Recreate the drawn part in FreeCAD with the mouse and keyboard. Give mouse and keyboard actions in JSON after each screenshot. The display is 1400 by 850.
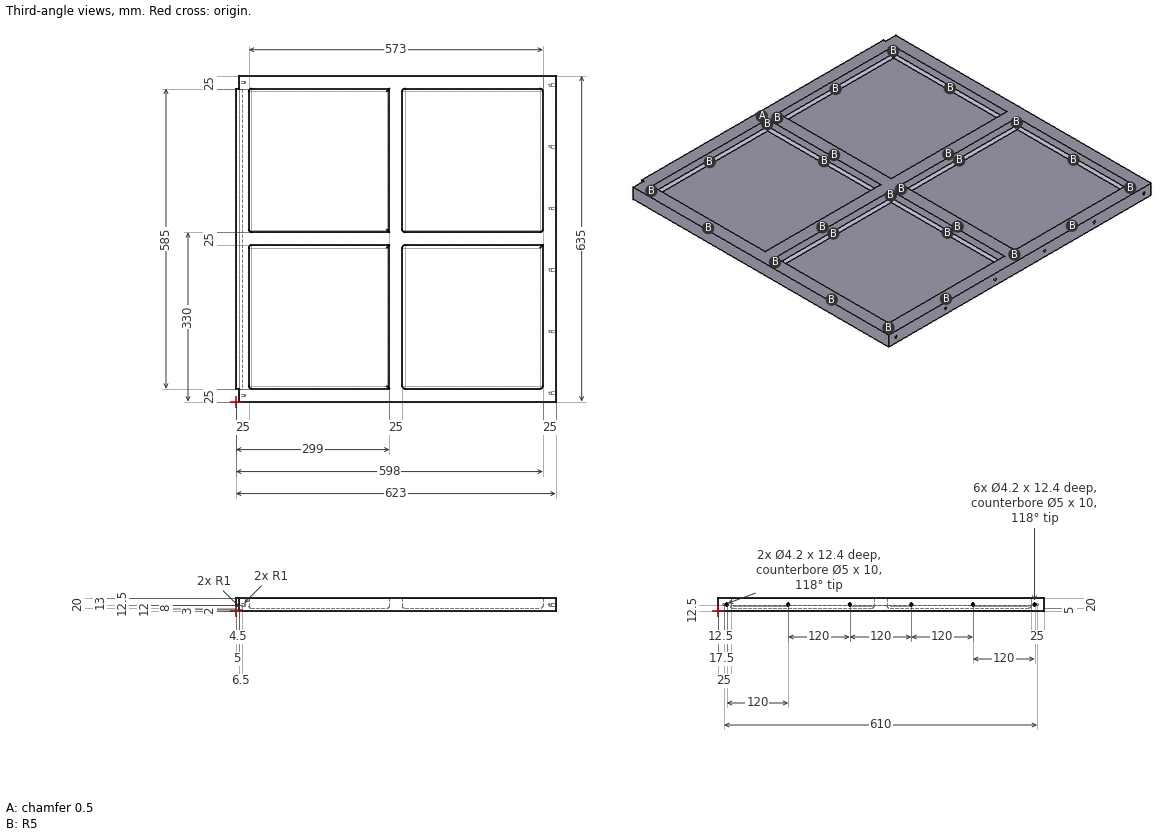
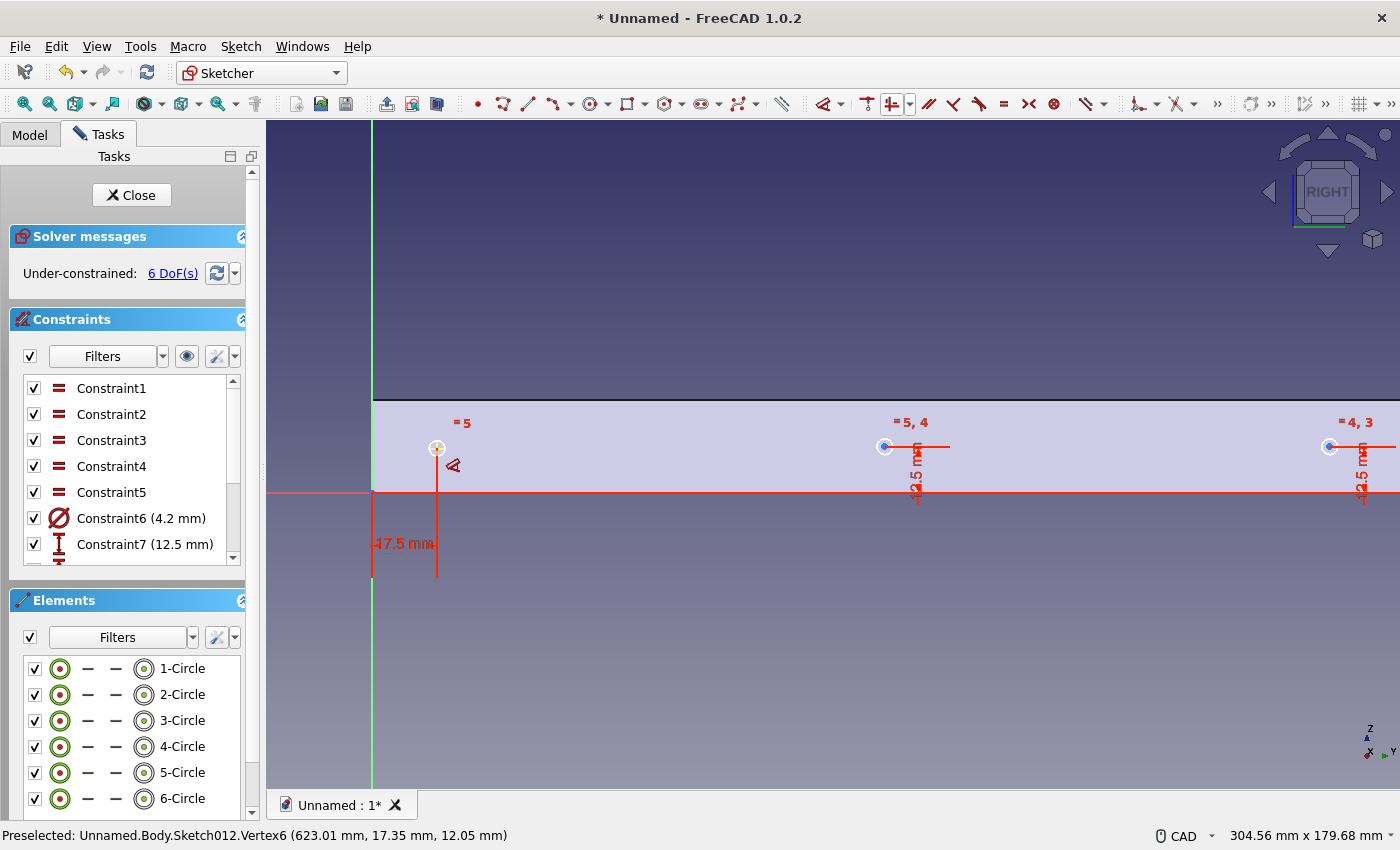
{"action": "left_click", "coordinate": [437, 448]}
{"action": "left_click", "coordinate": [338, 471]}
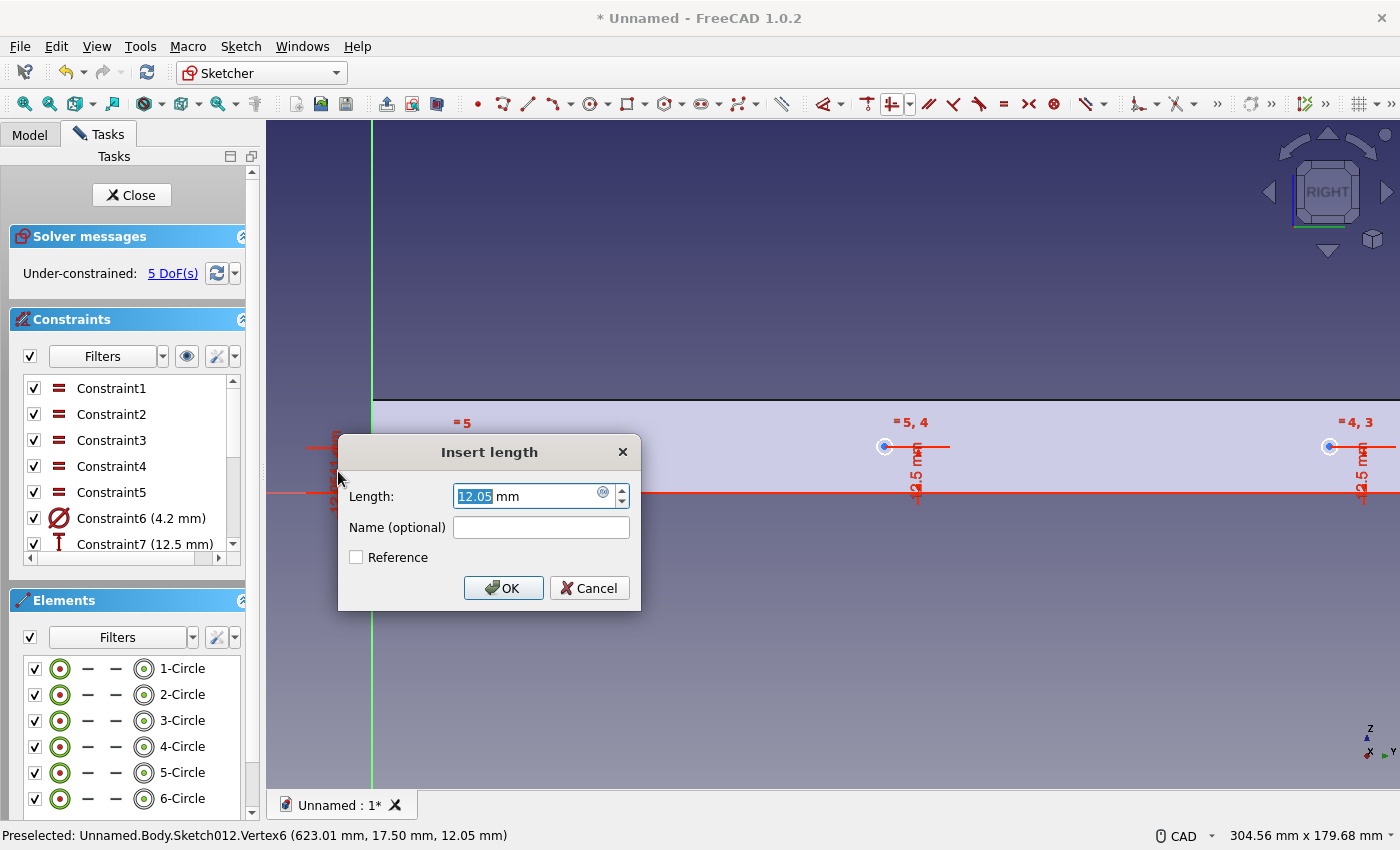
{"action": "type", "text": "12.5"}
{"action": "key", "text": "Return"}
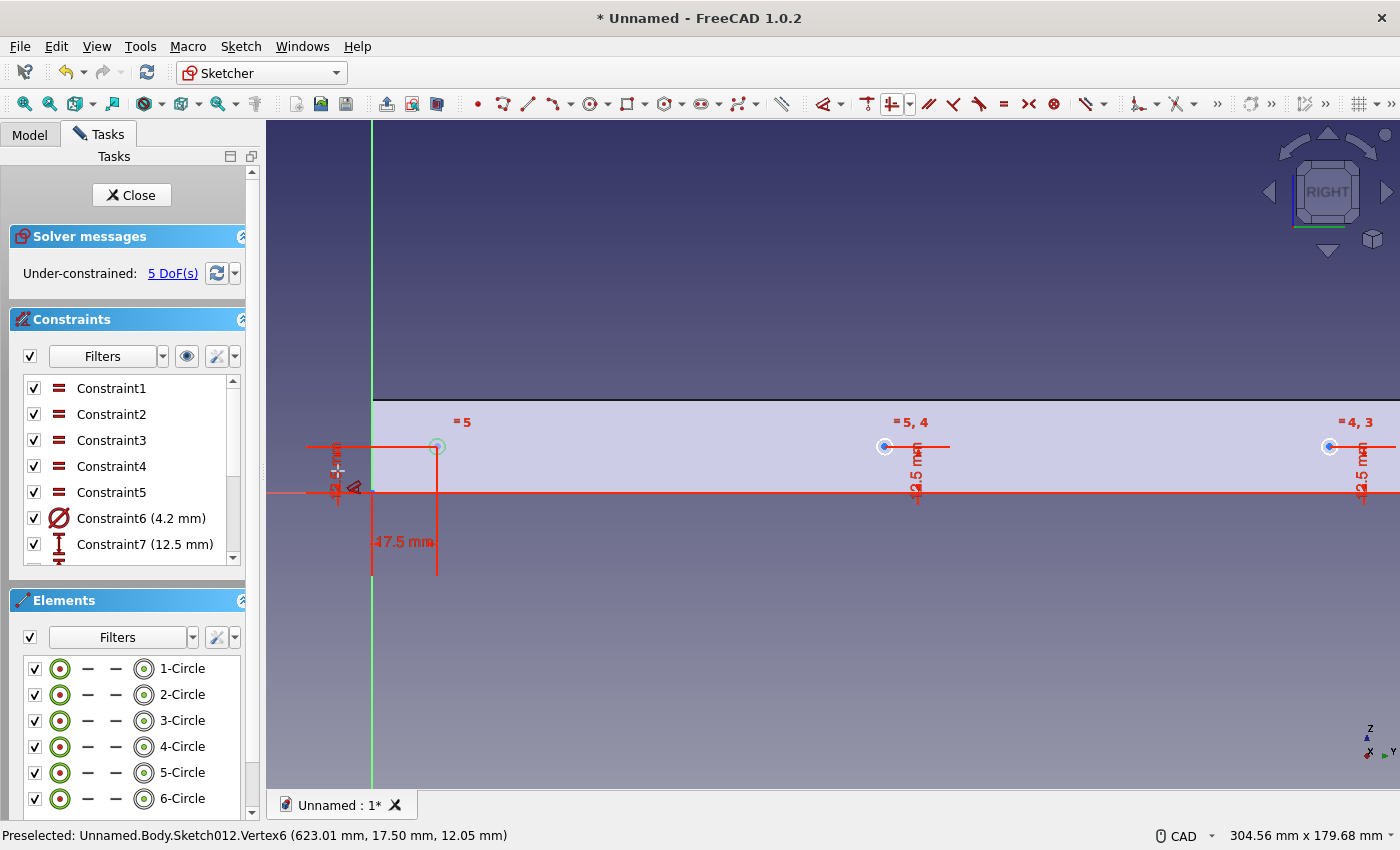
{"action": "scroll", "coordinate": [436, 449], "scroll_direction": "down", "scroll_amount": 6}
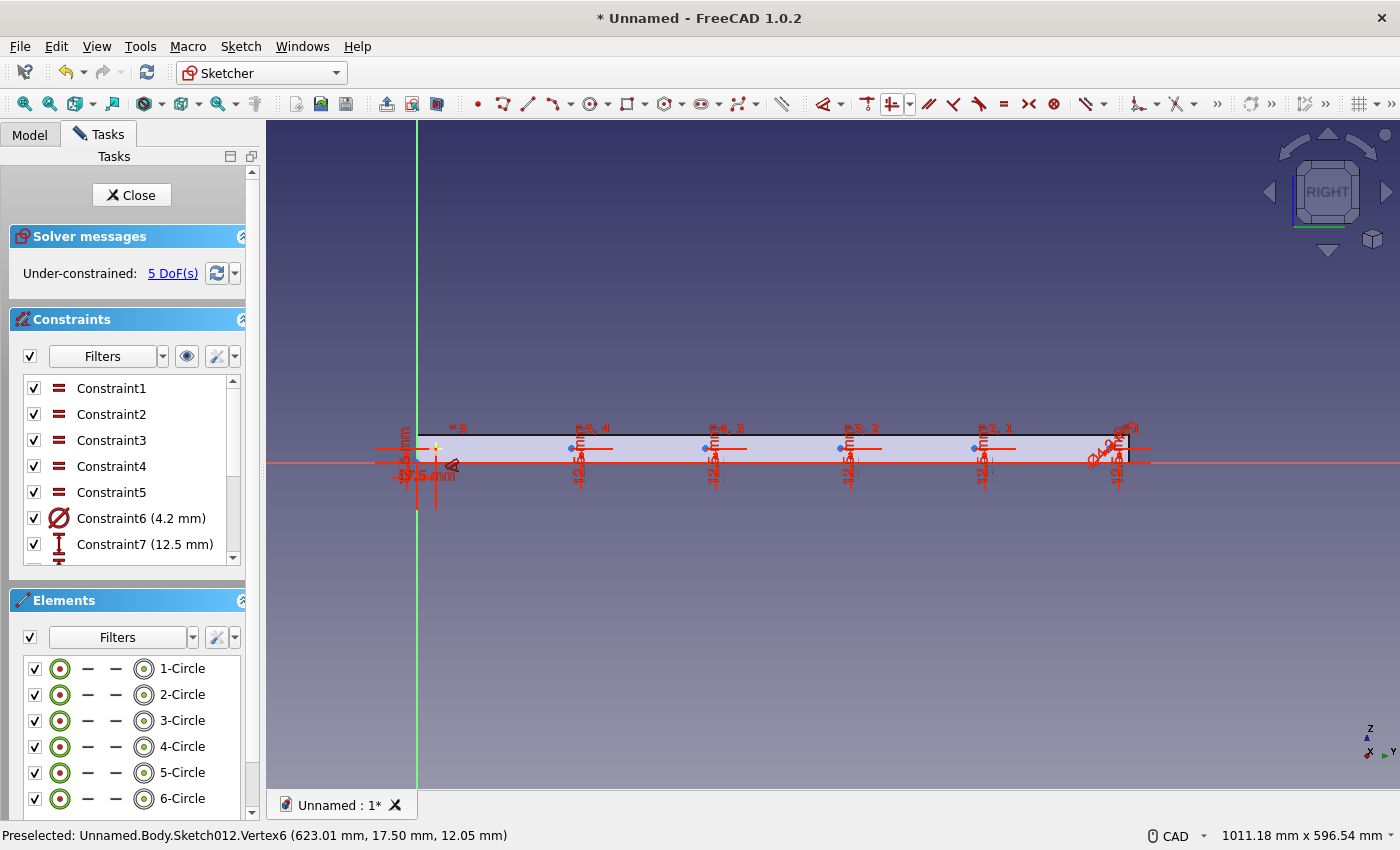
{"action": "left_click", "coordinate": [1109, 449]}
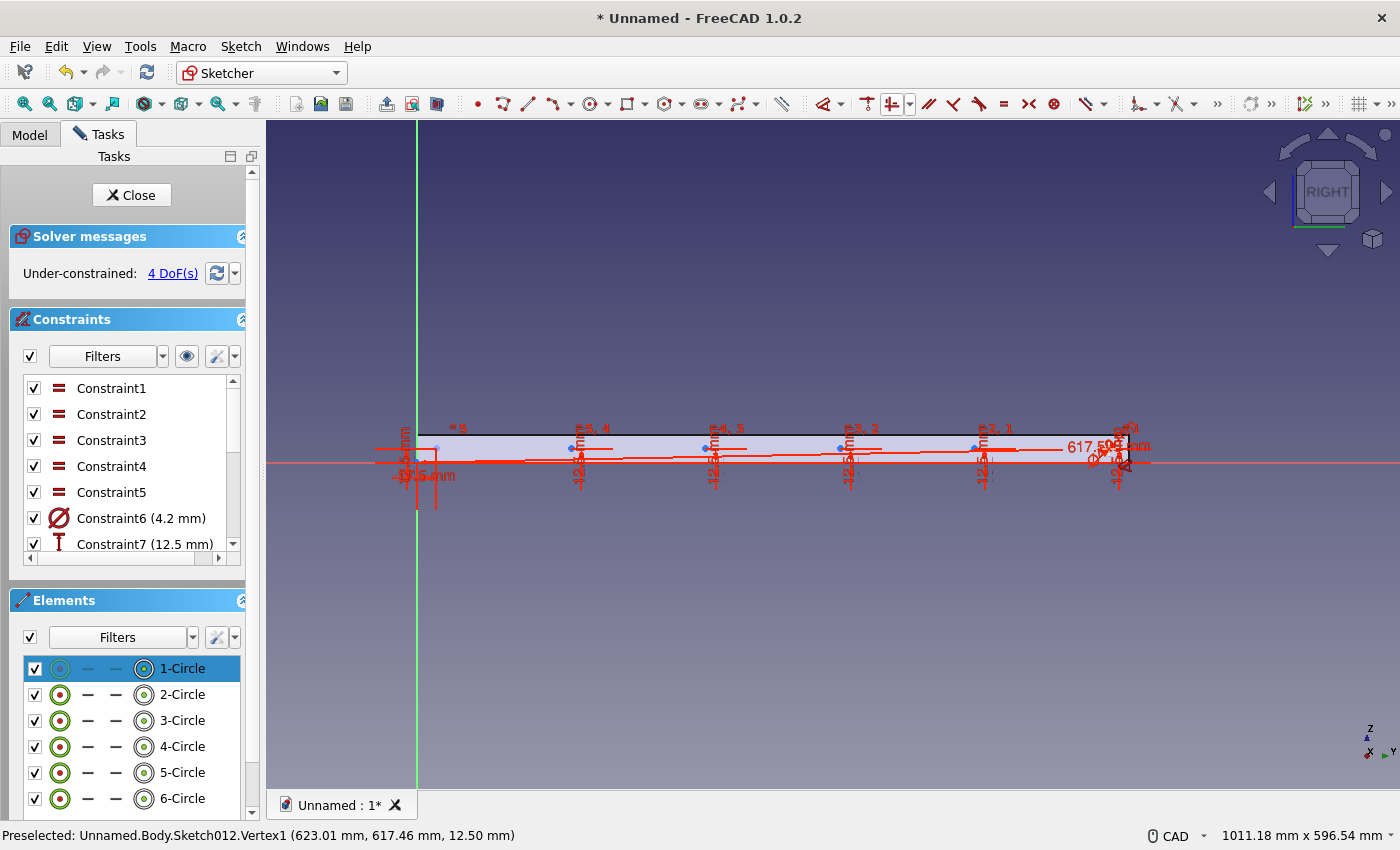
{"action": "left_click", "coordinate": [974, 449]}
{"action": "left_click", "coordinate": [1042, 415]}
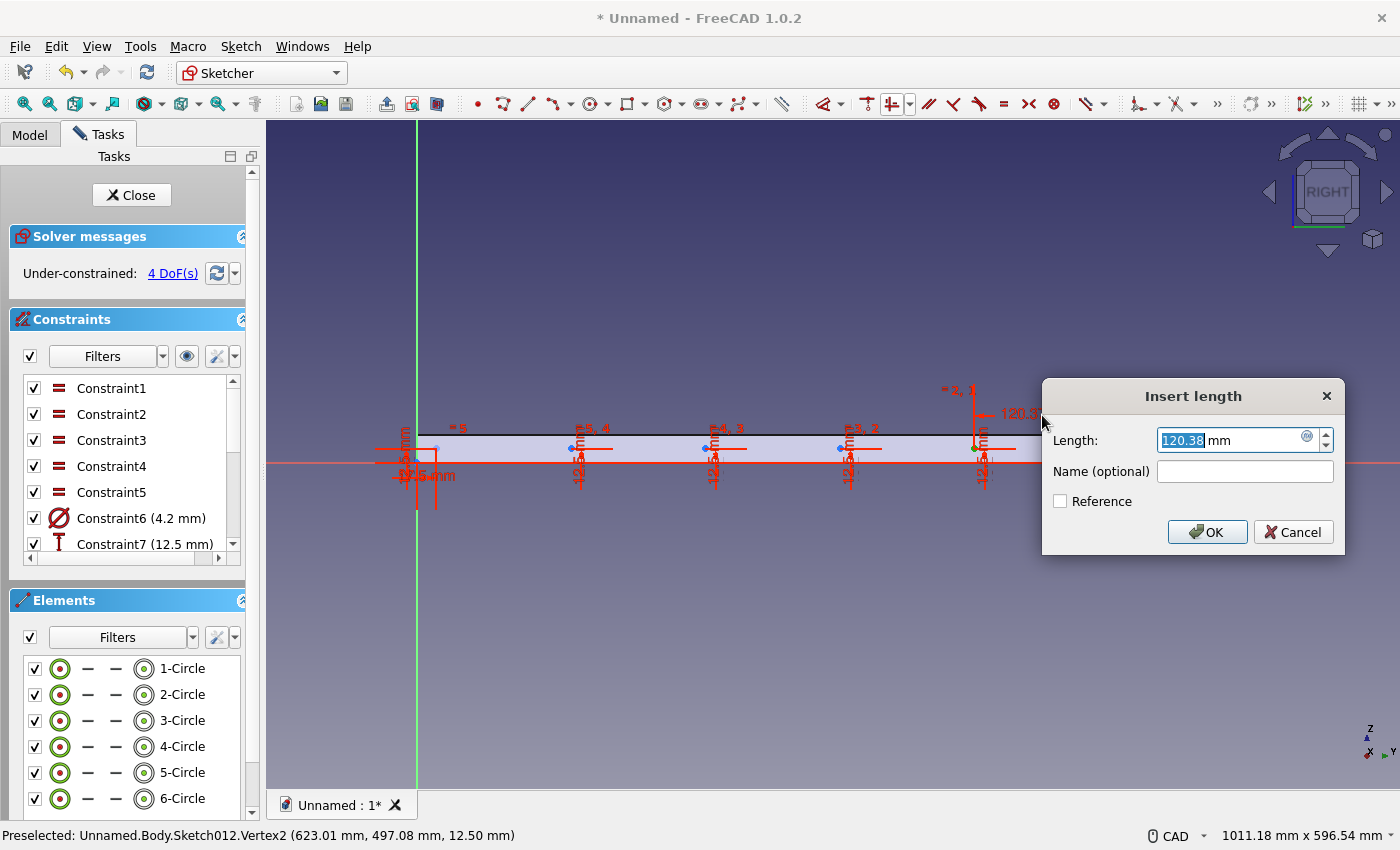
{"action": "type", "text": "120"}
{"action": "key", "text": "Return"}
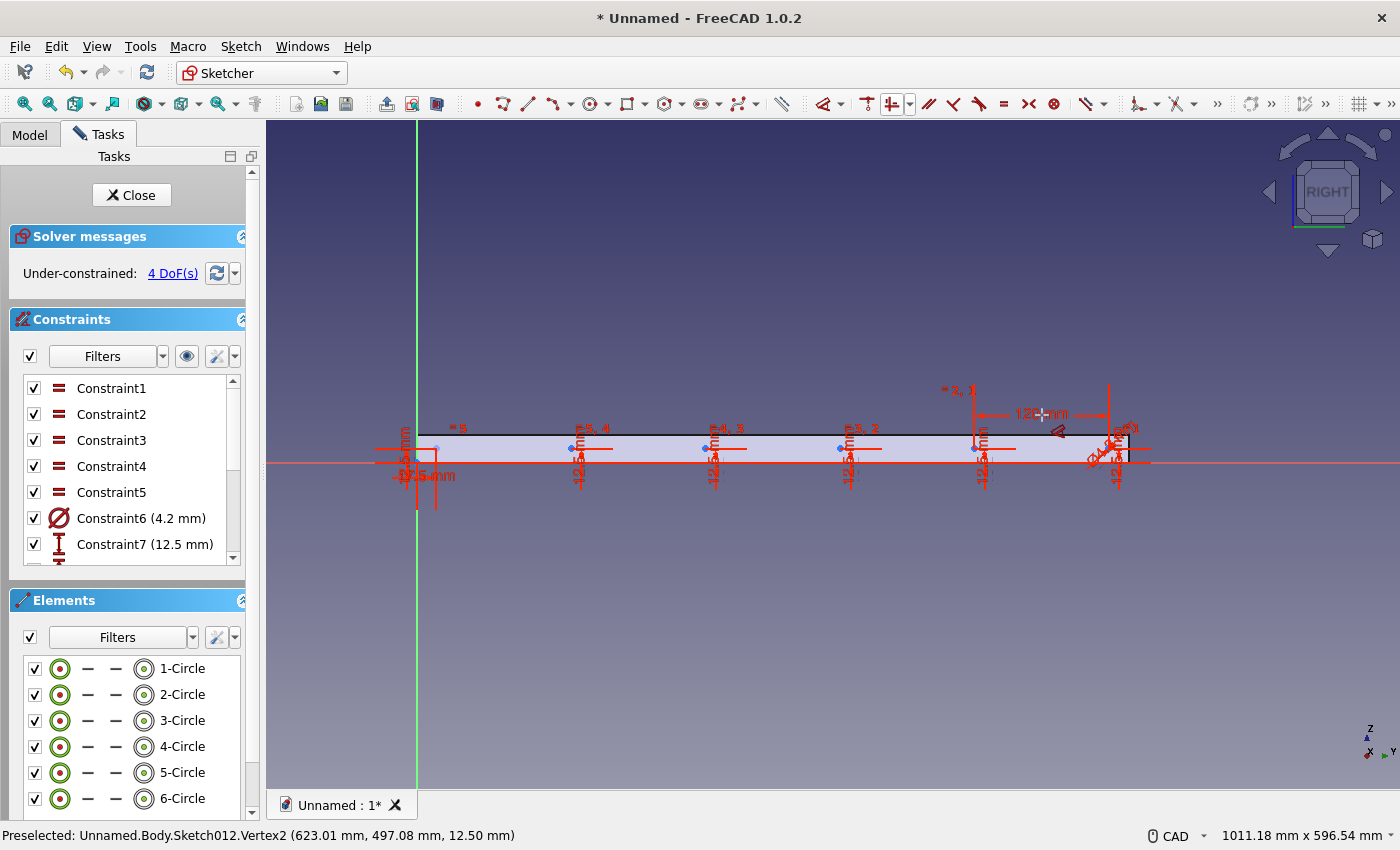
{"action": "left_click", "coordinate": [974, 449]}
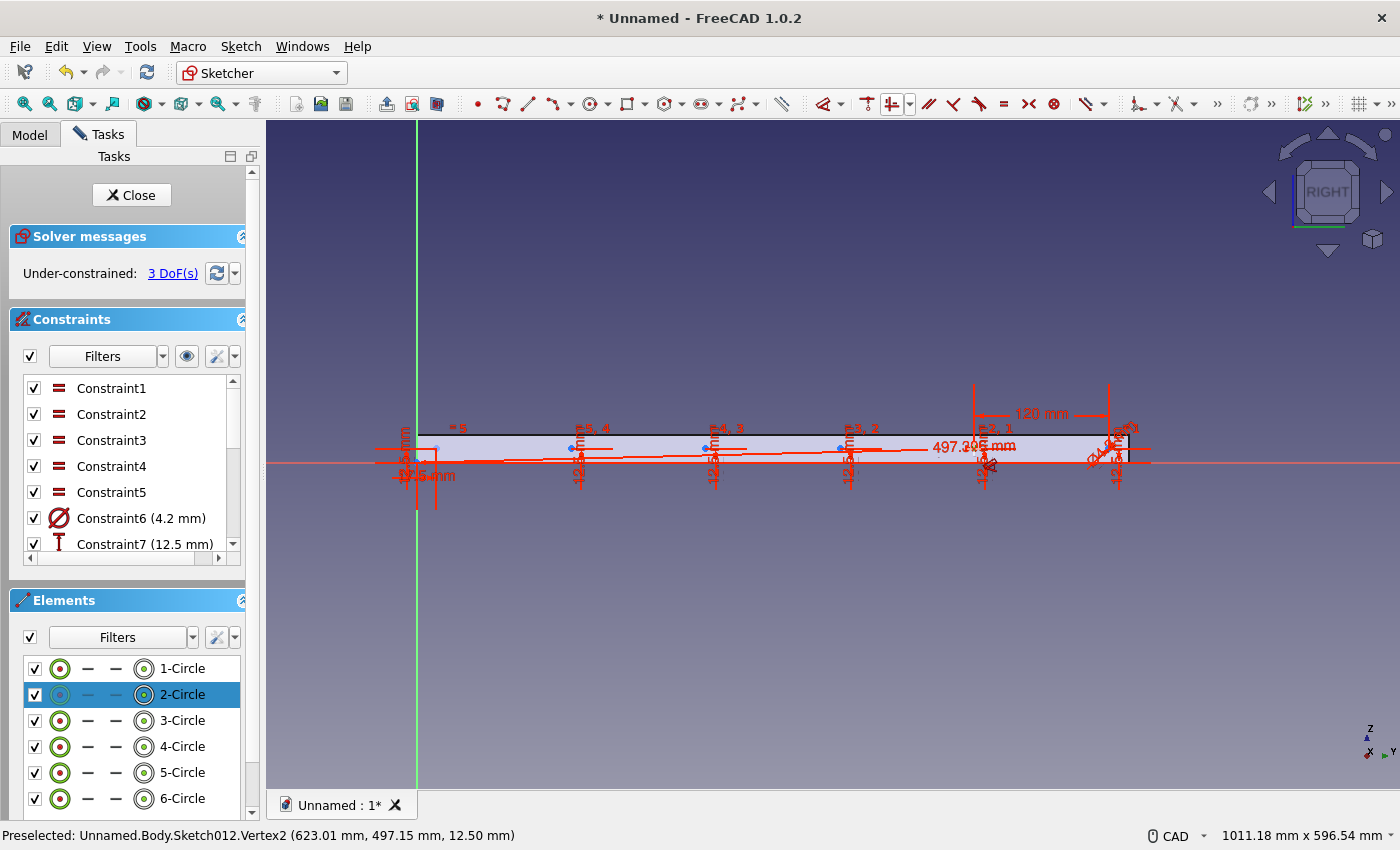
{"action": "left_click", "coordinate": [840, 449]}
{"action": "left_click", "coordinate": [907, 415]}